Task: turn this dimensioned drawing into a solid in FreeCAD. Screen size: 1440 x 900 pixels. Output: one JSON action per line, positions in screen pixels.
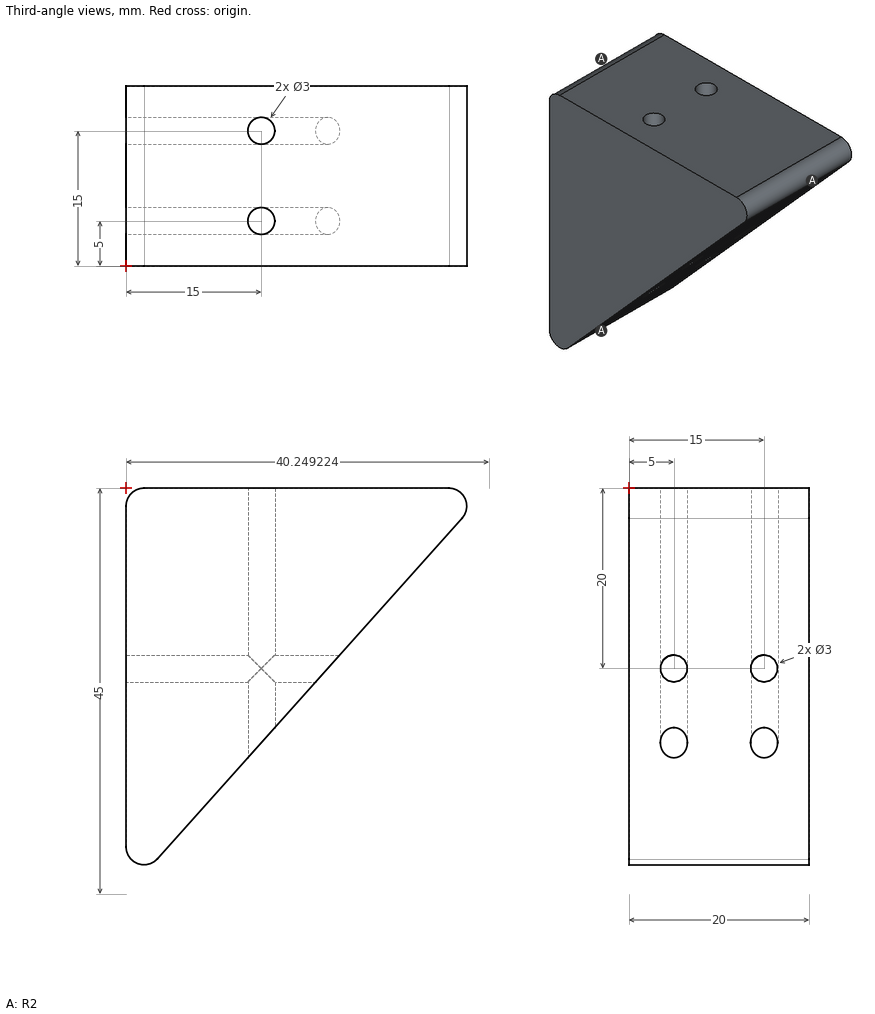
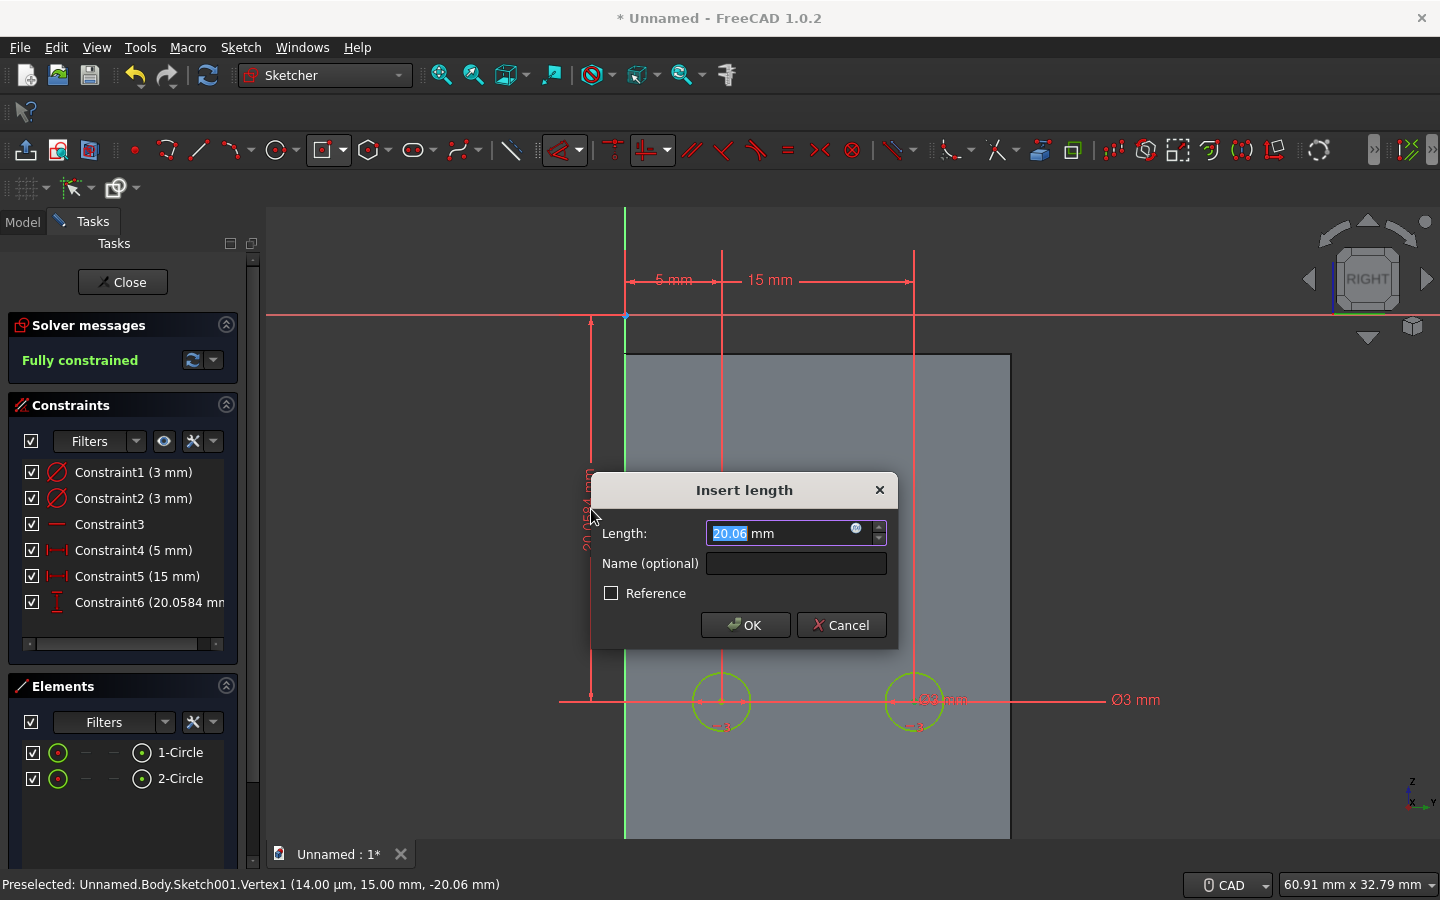
{"action": "type", "text": "20"}
{"action": "key", "text": "Return"}
{"action": "key", "text": "Escape"}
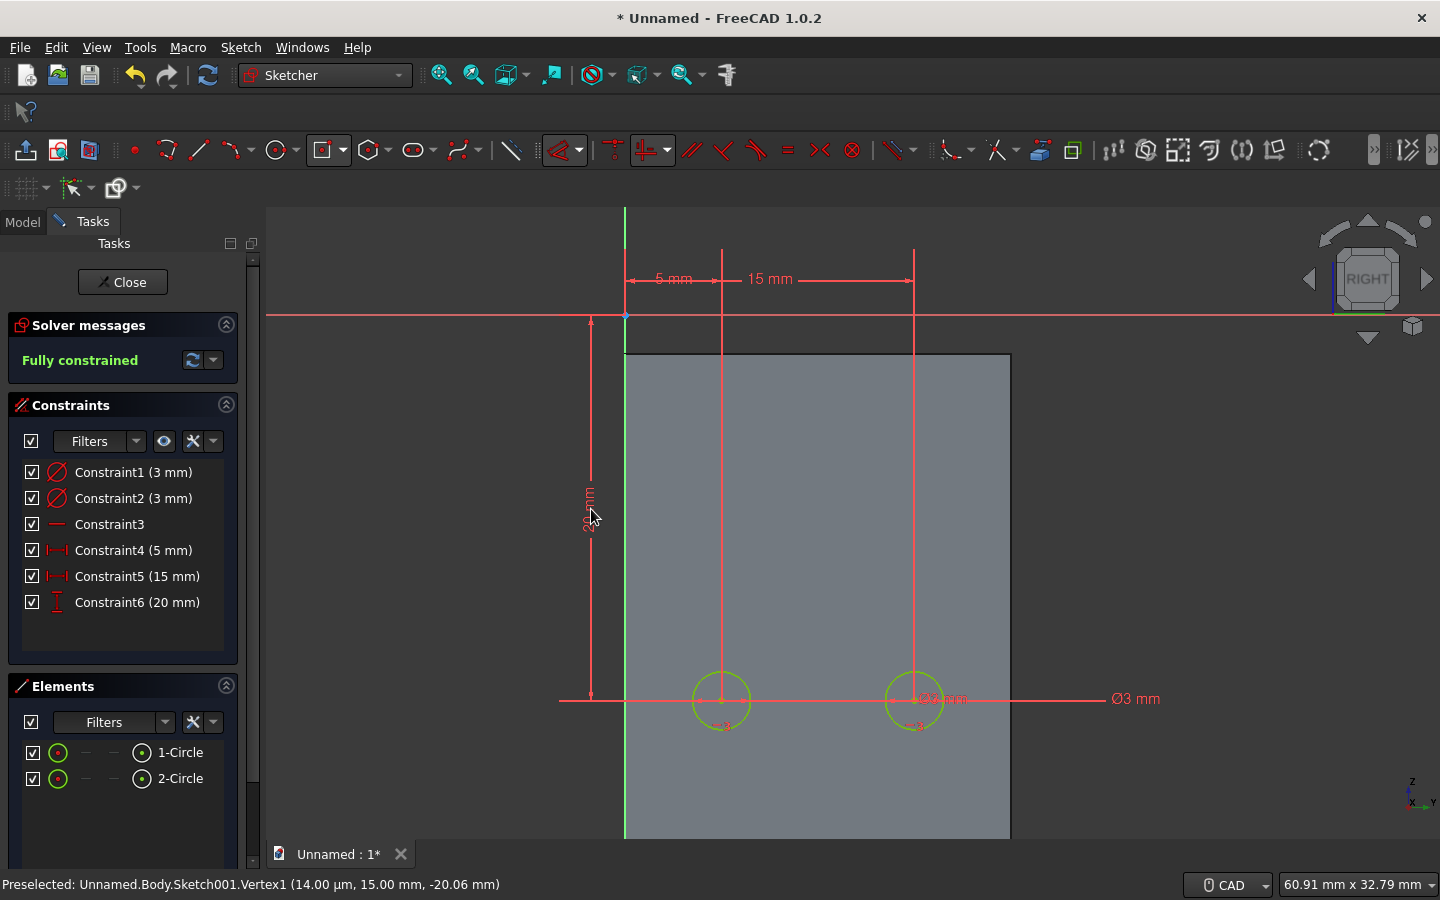
{"action": "left_click", "coordinate": [123, 282]}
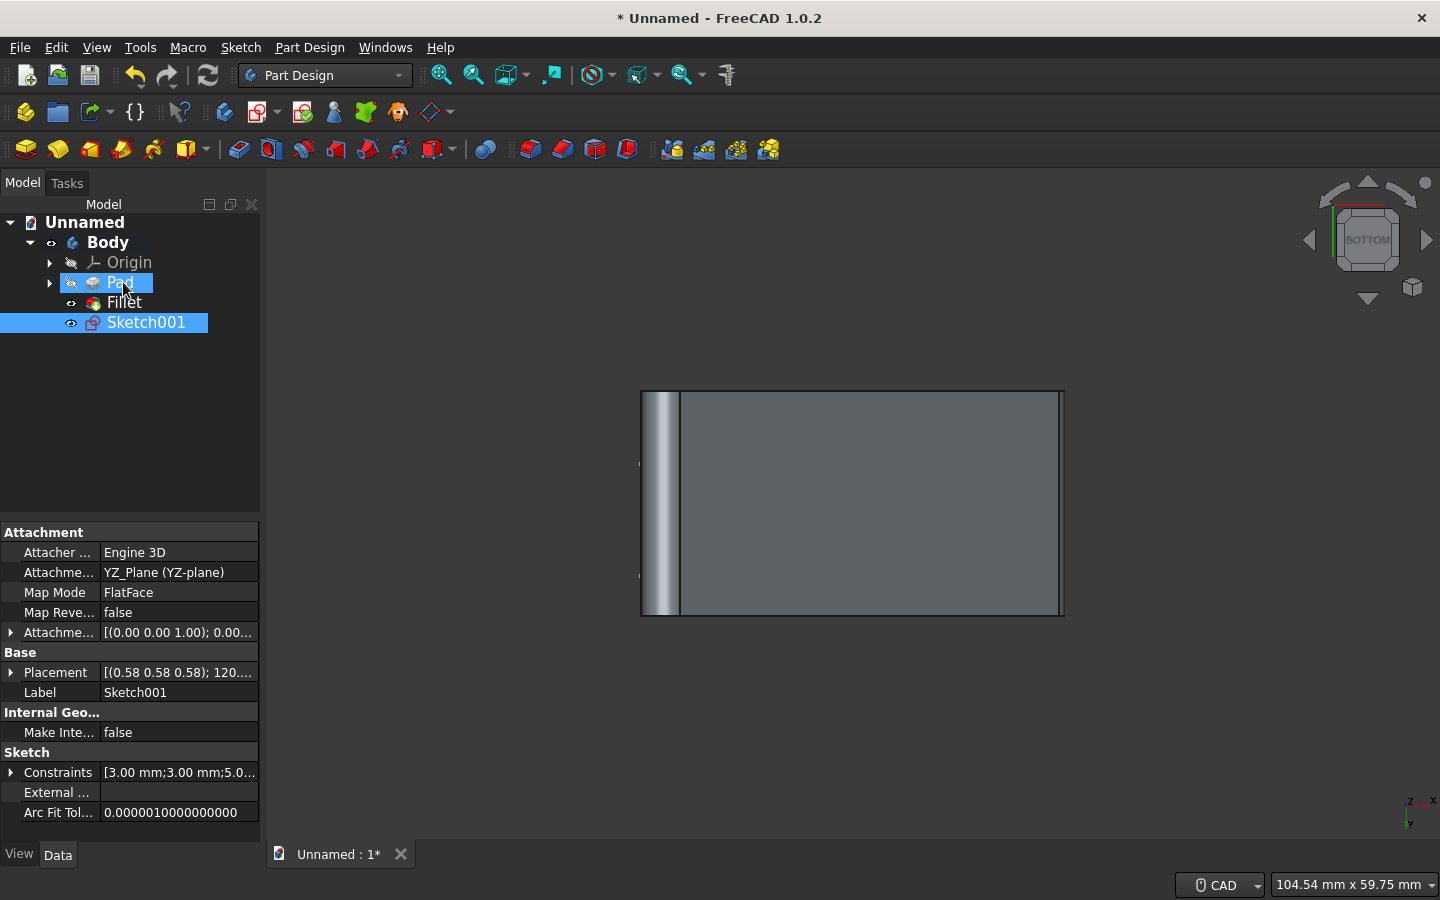
{"action": "left_click", "coordinate": [240, 150]}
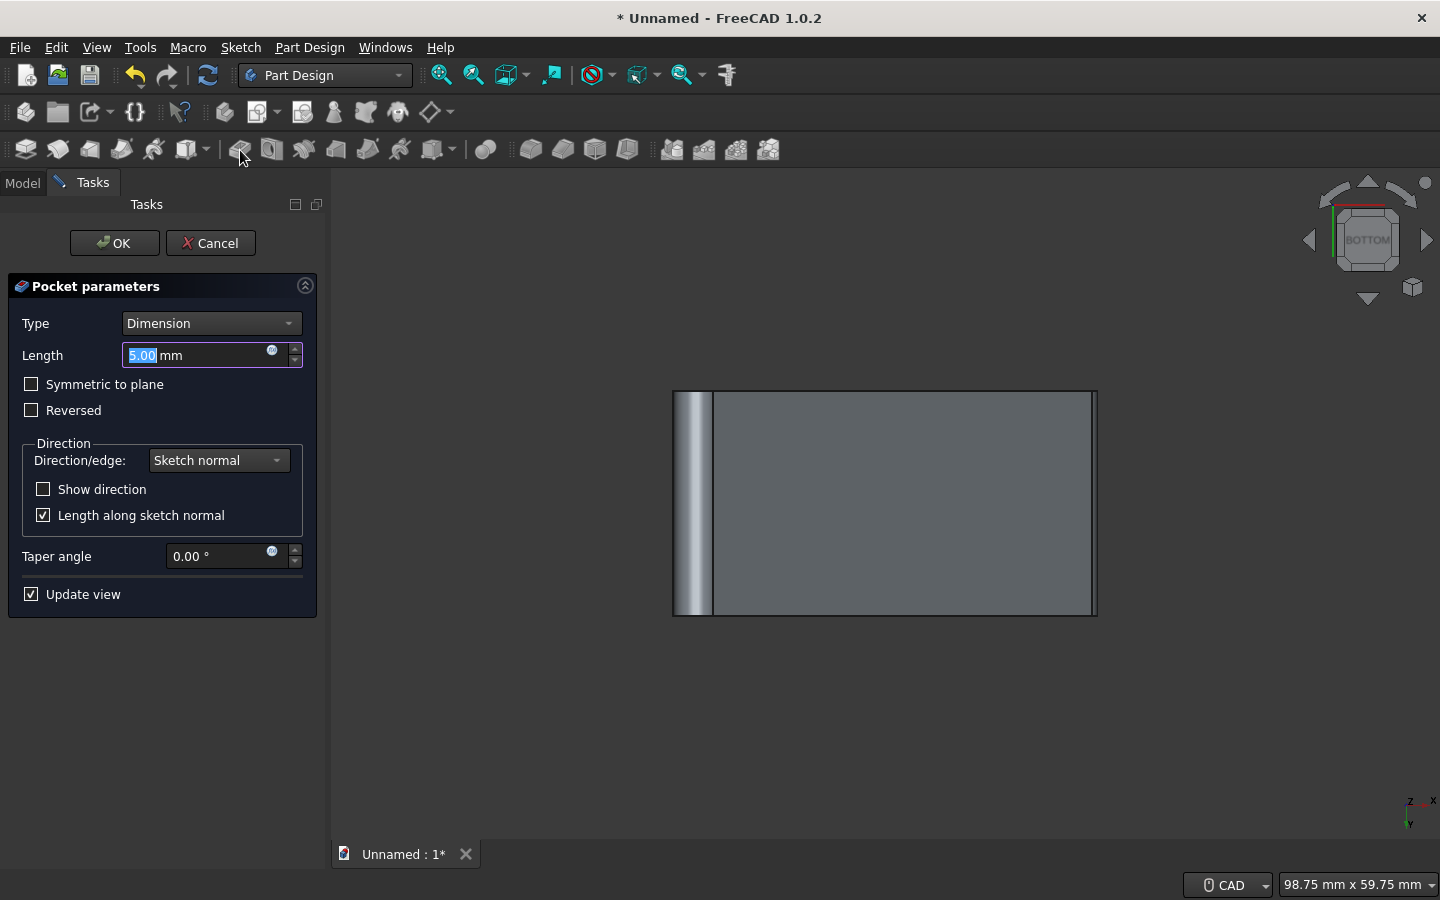
{"action": "left_click", "coordinate": [212, 324]}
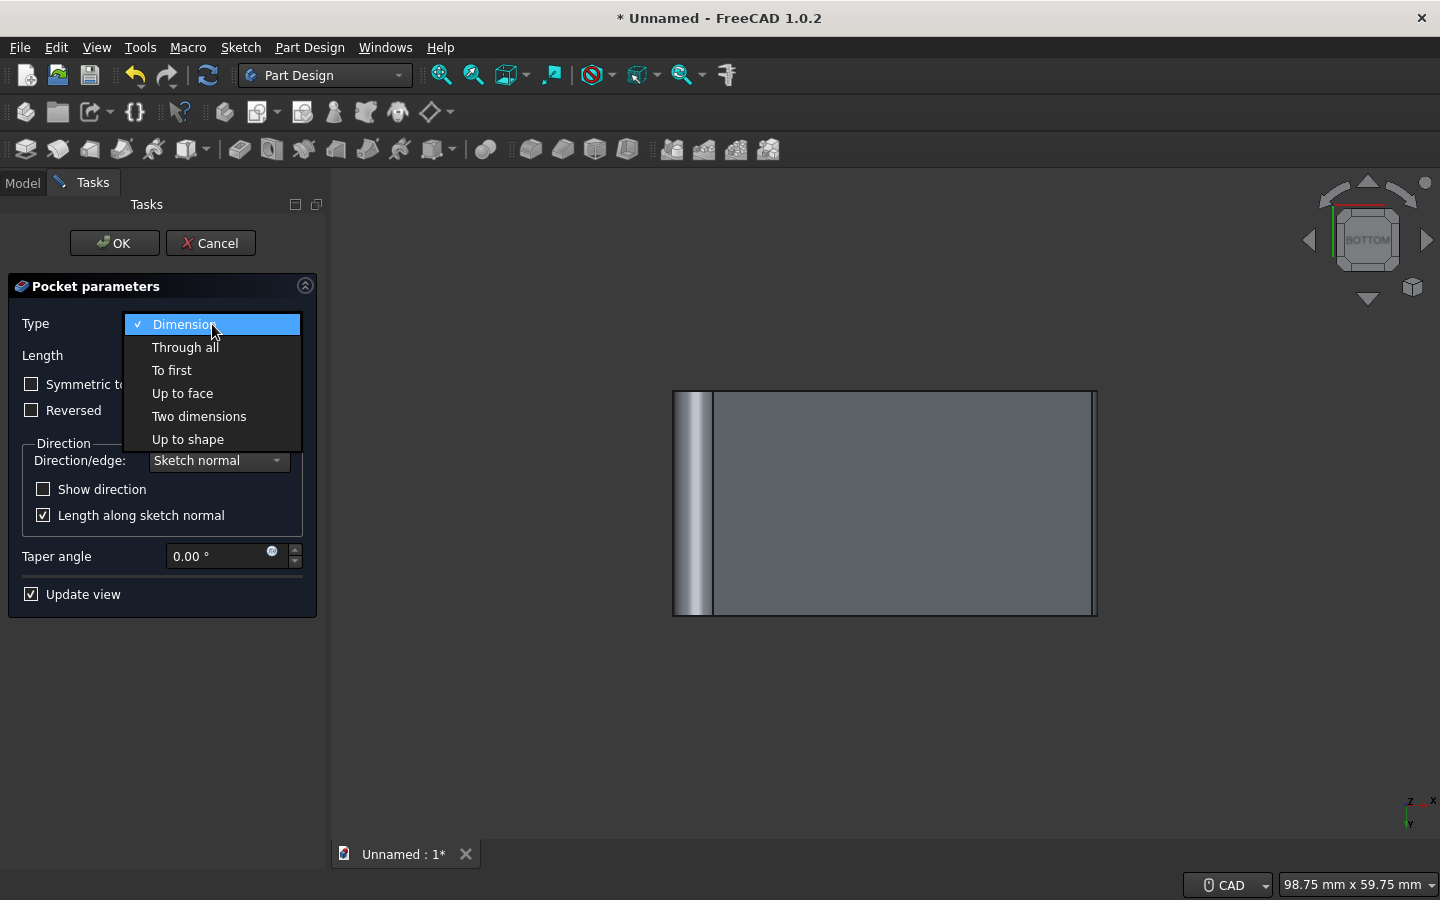
{"action": "left_click", "coordinate": [212, 348]}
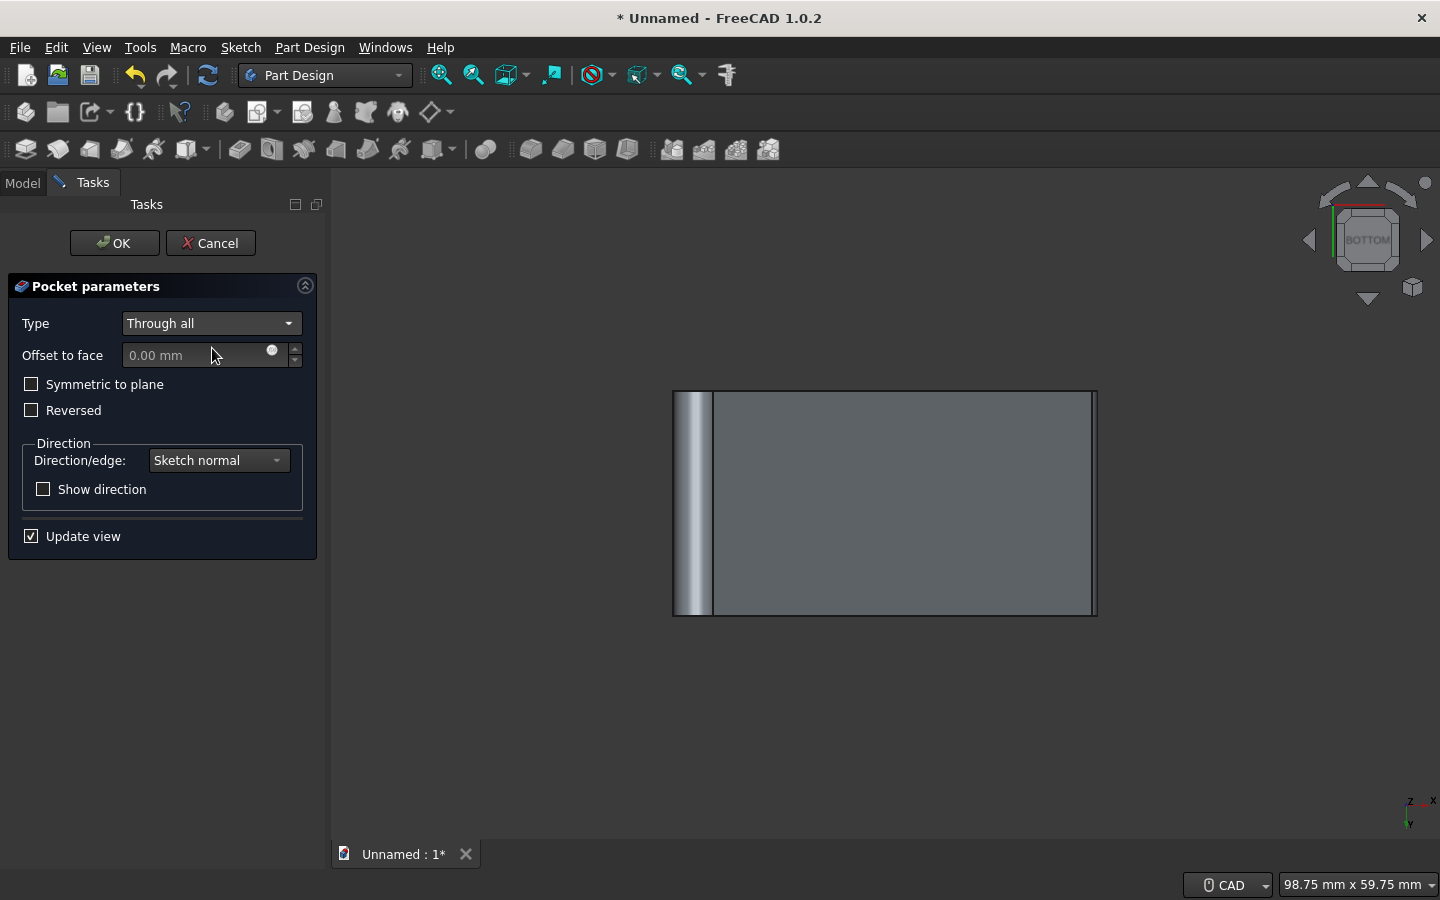
{"action": "left_click", "coordinate": [30, 410]}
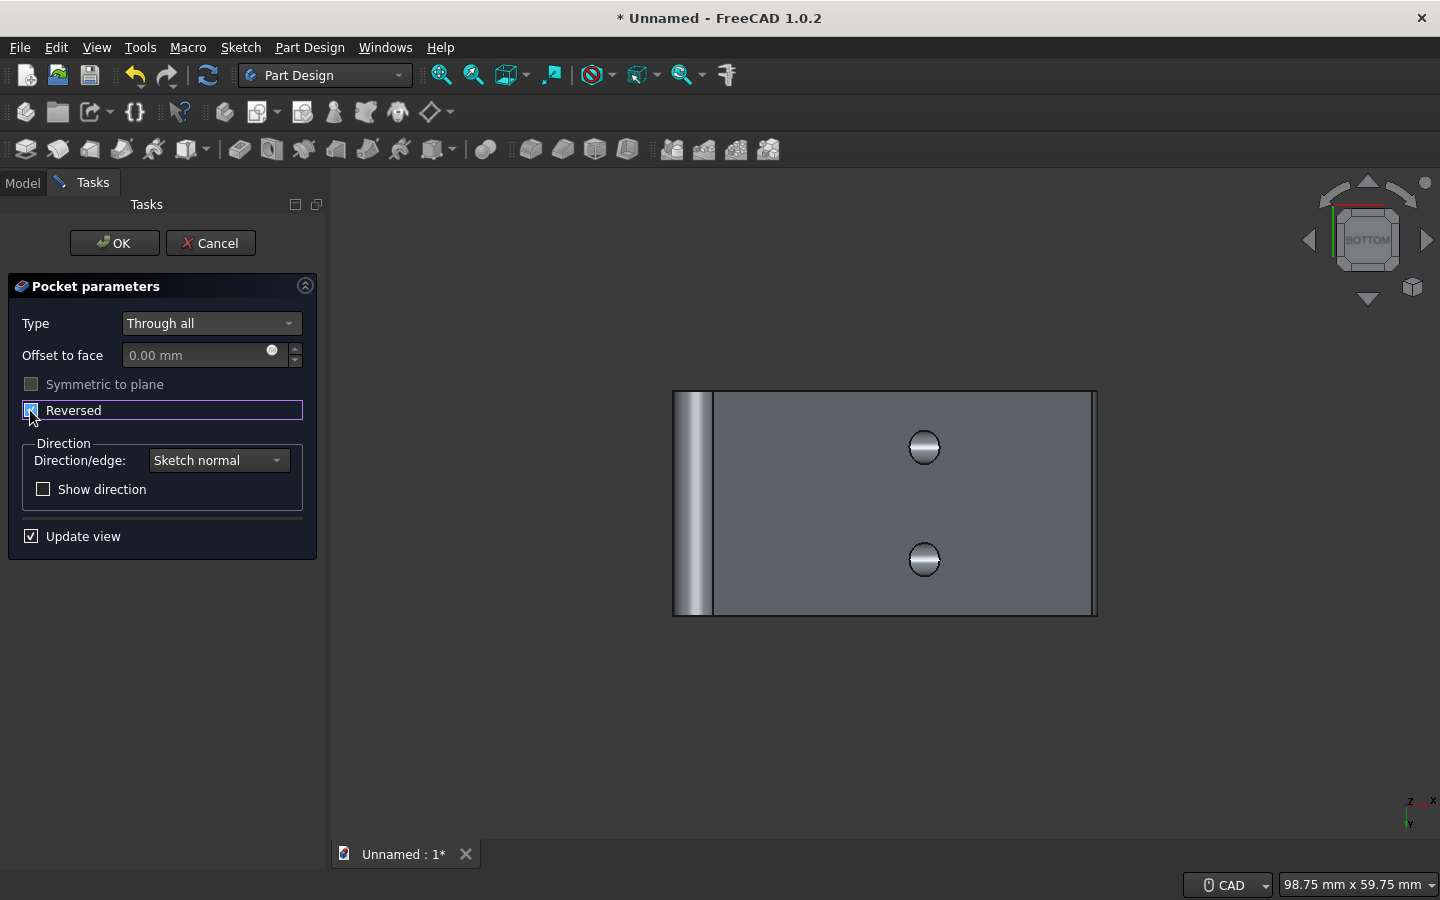
{"action": "left_click", "coordinate": [115, 243]}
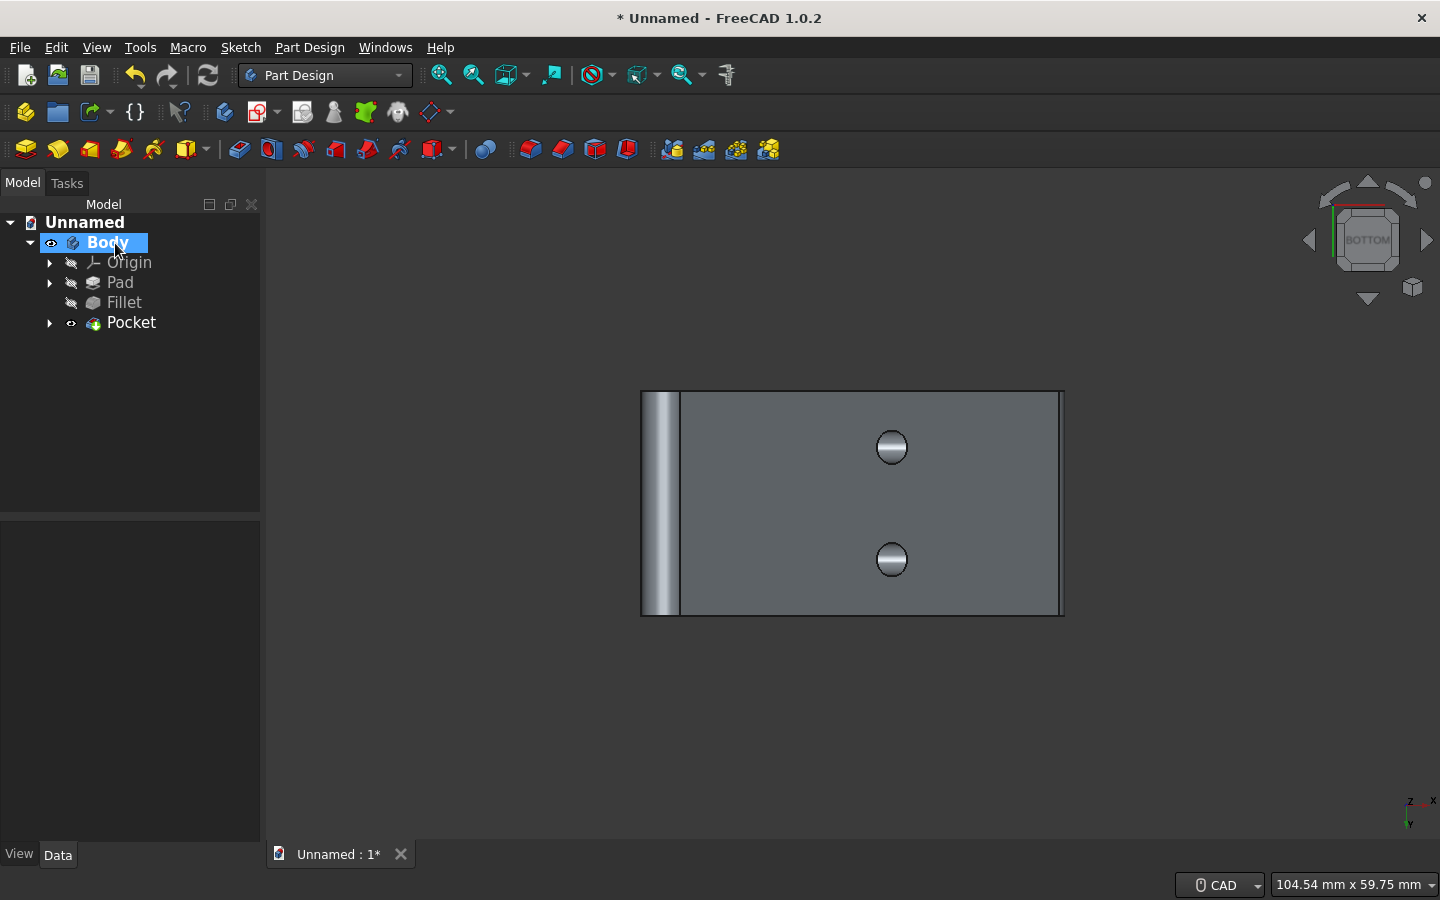
{"action": "key", "text": "v f"}